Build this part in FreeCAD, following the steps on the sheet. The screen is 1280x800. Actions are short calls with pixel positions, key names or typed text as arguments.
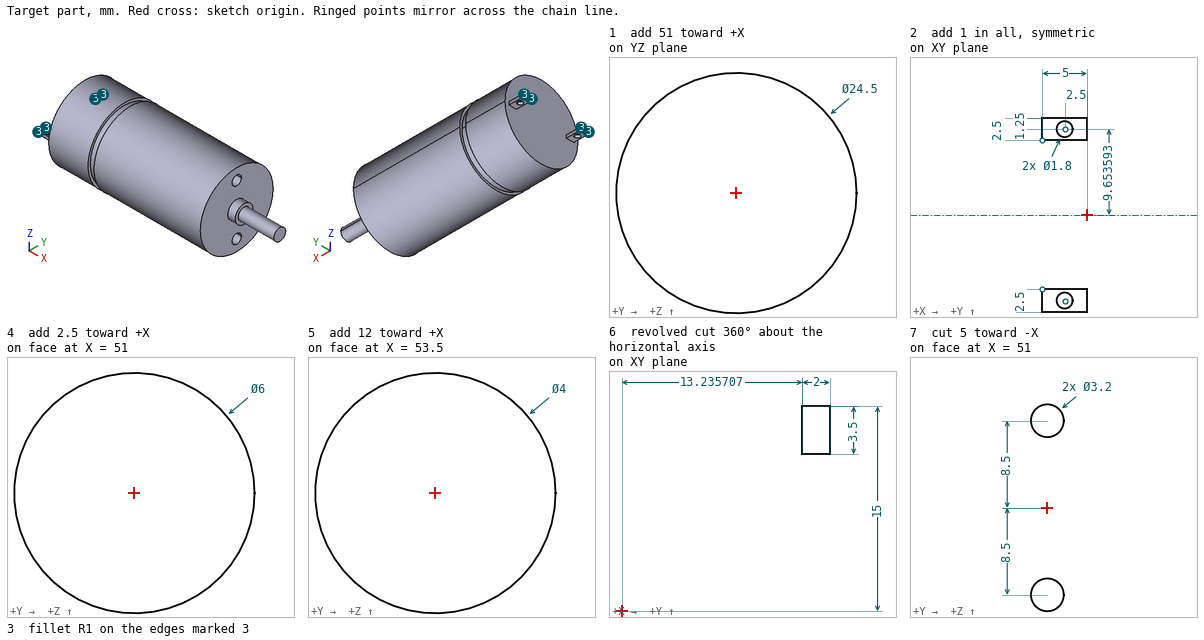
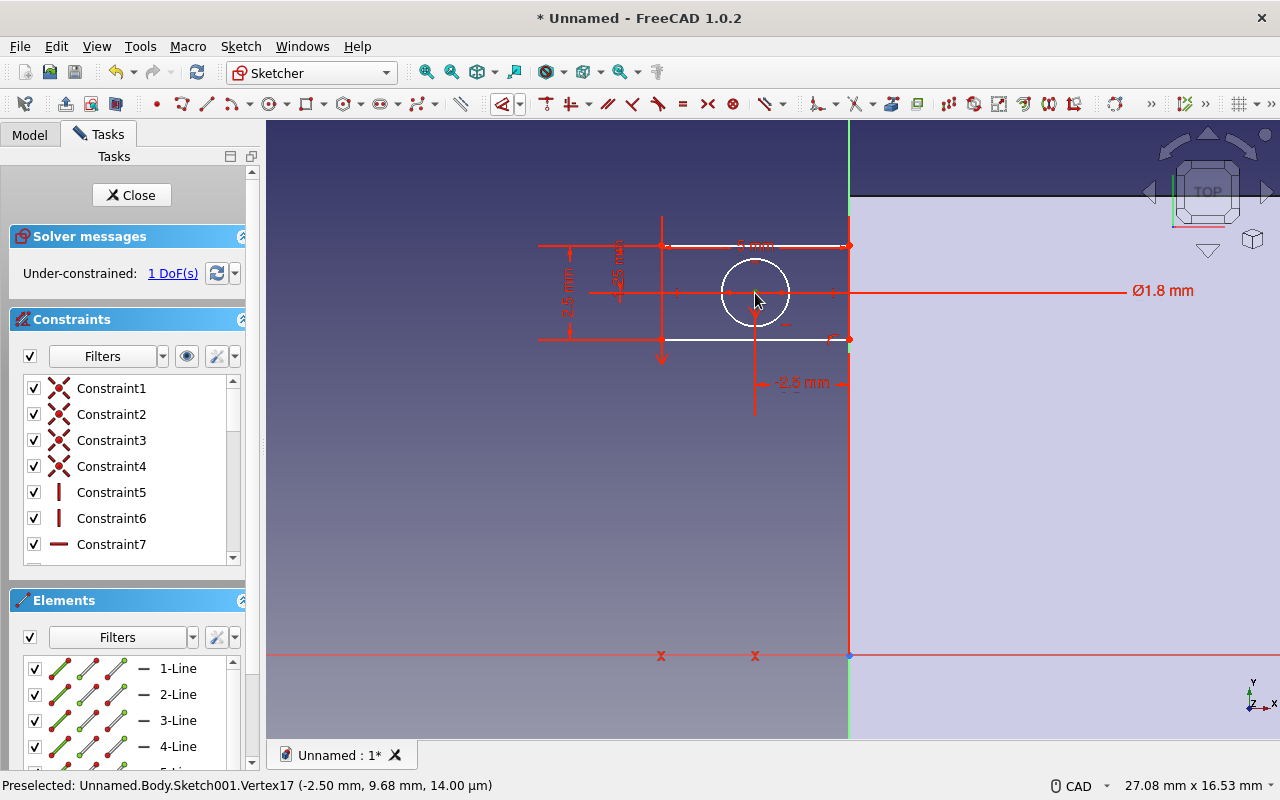
click(520, 104)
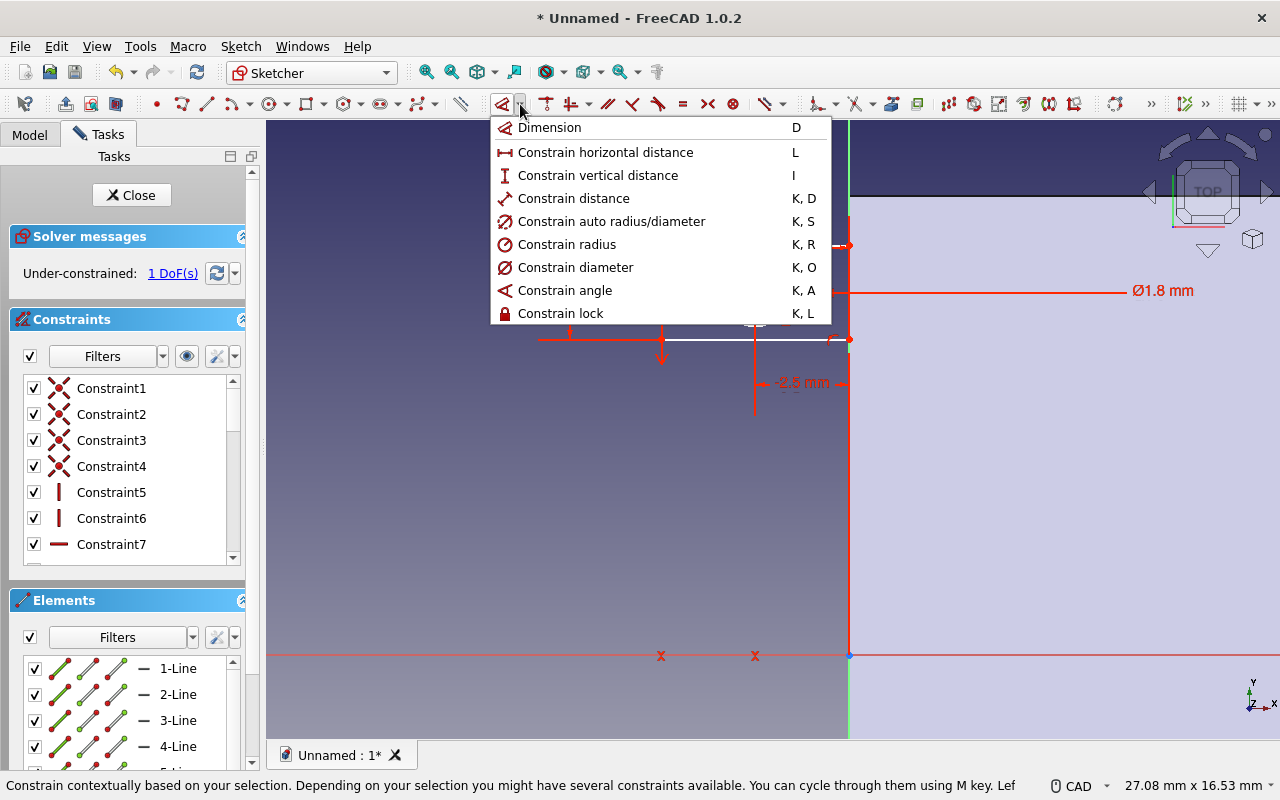
click(661, 176)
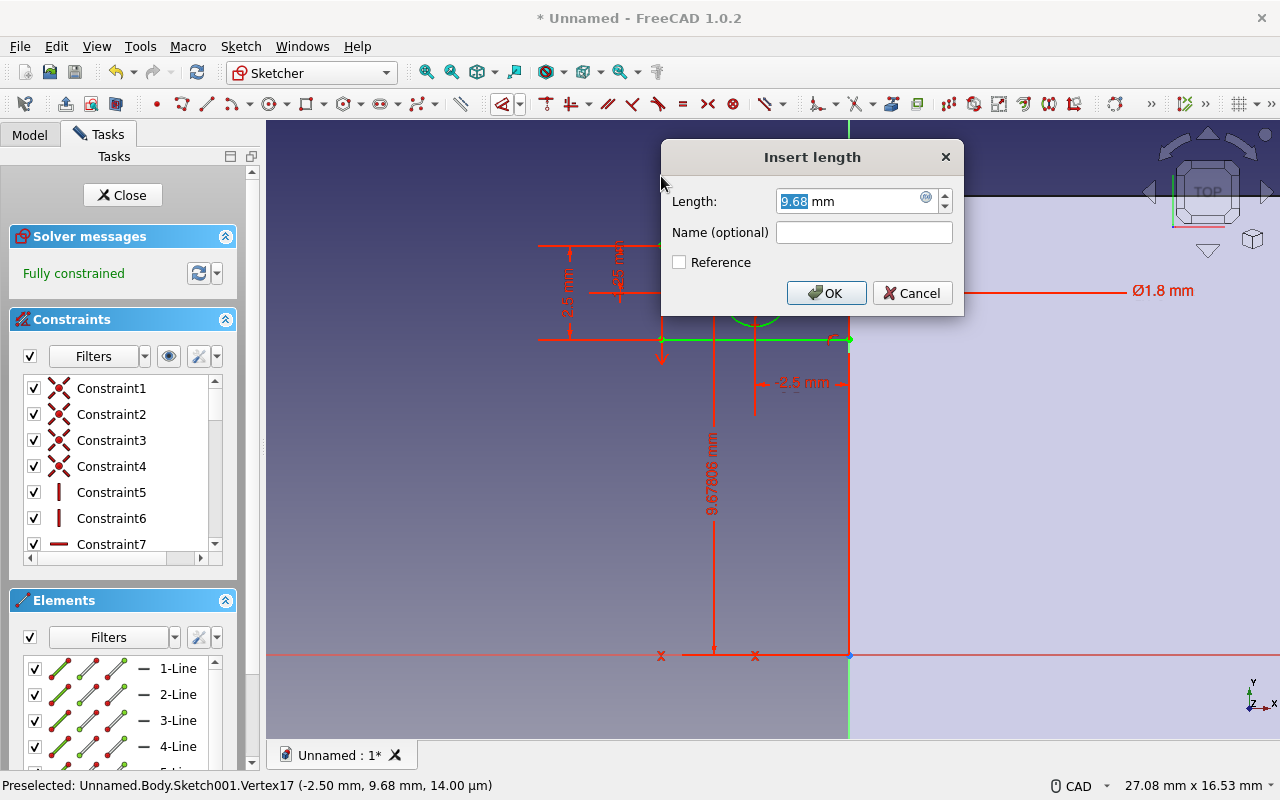
text(9.653593)
key(Return)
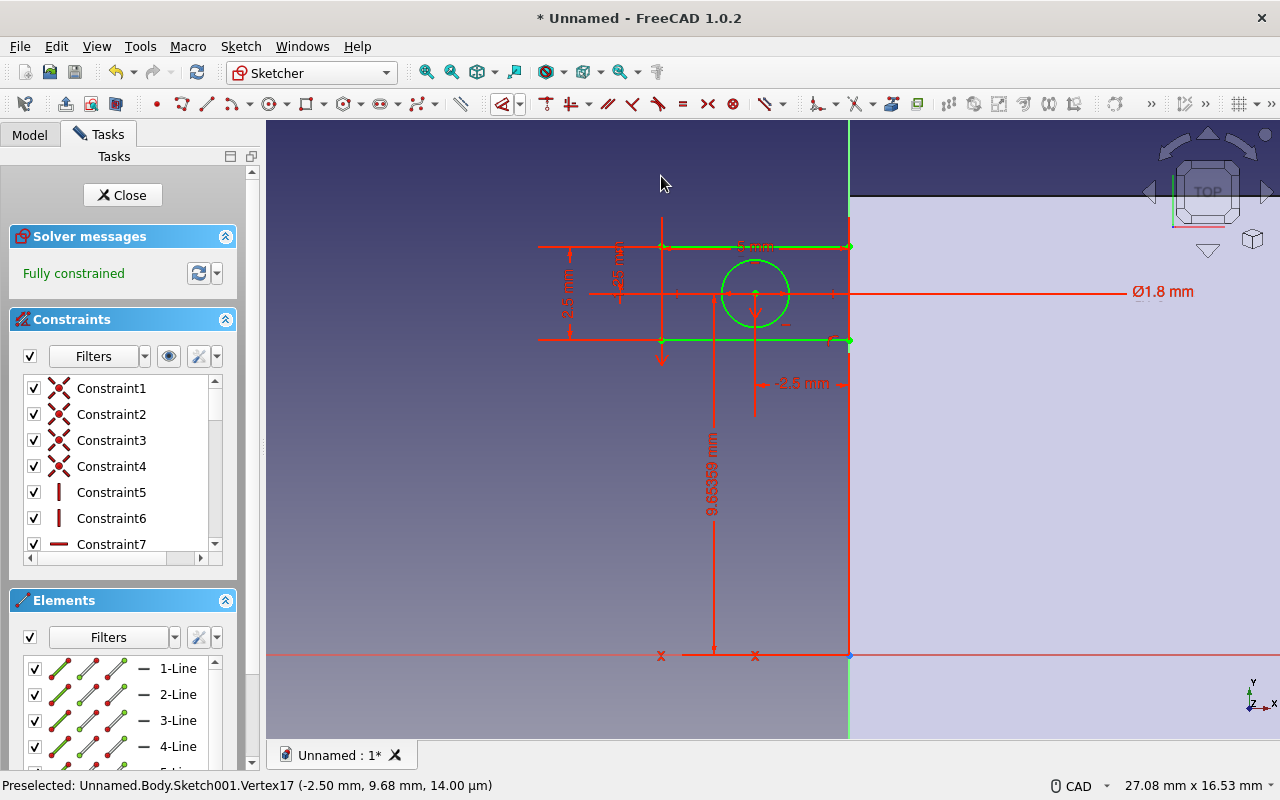
click(123, 195)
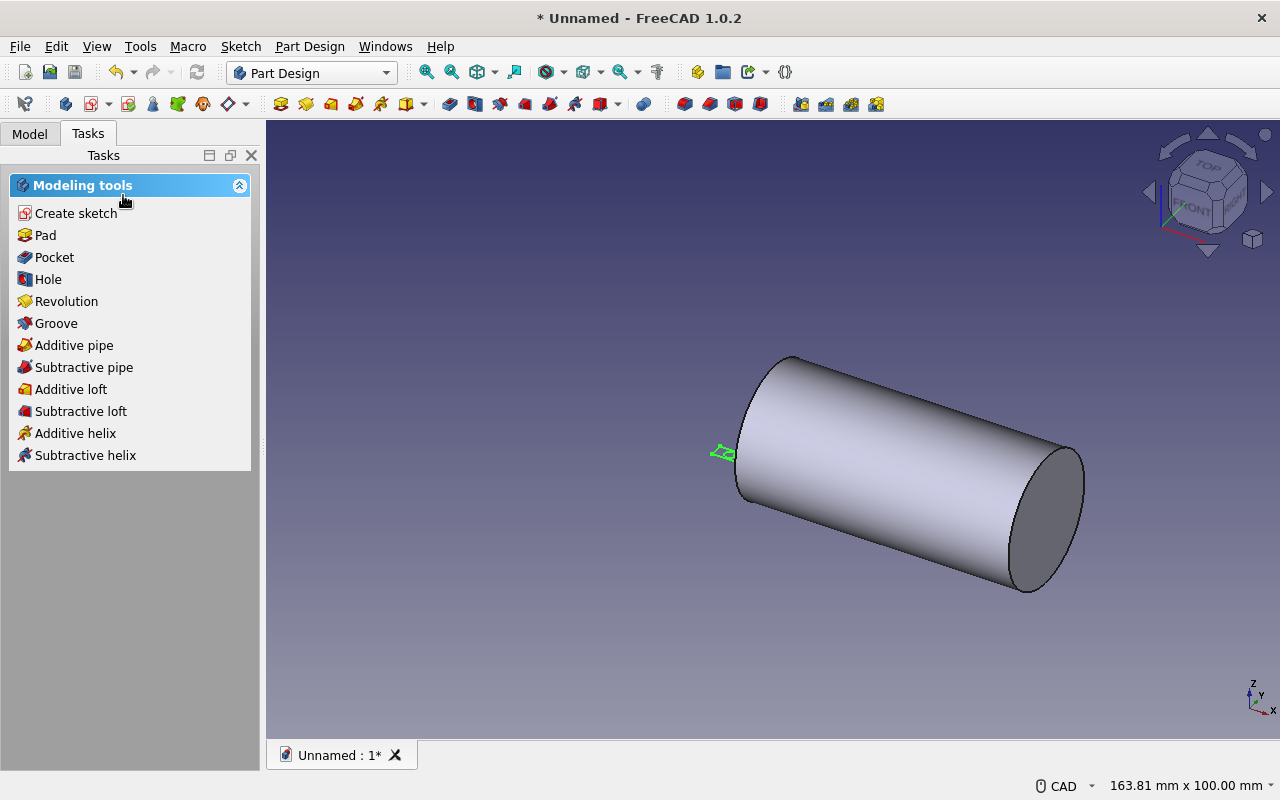
click(281, 104)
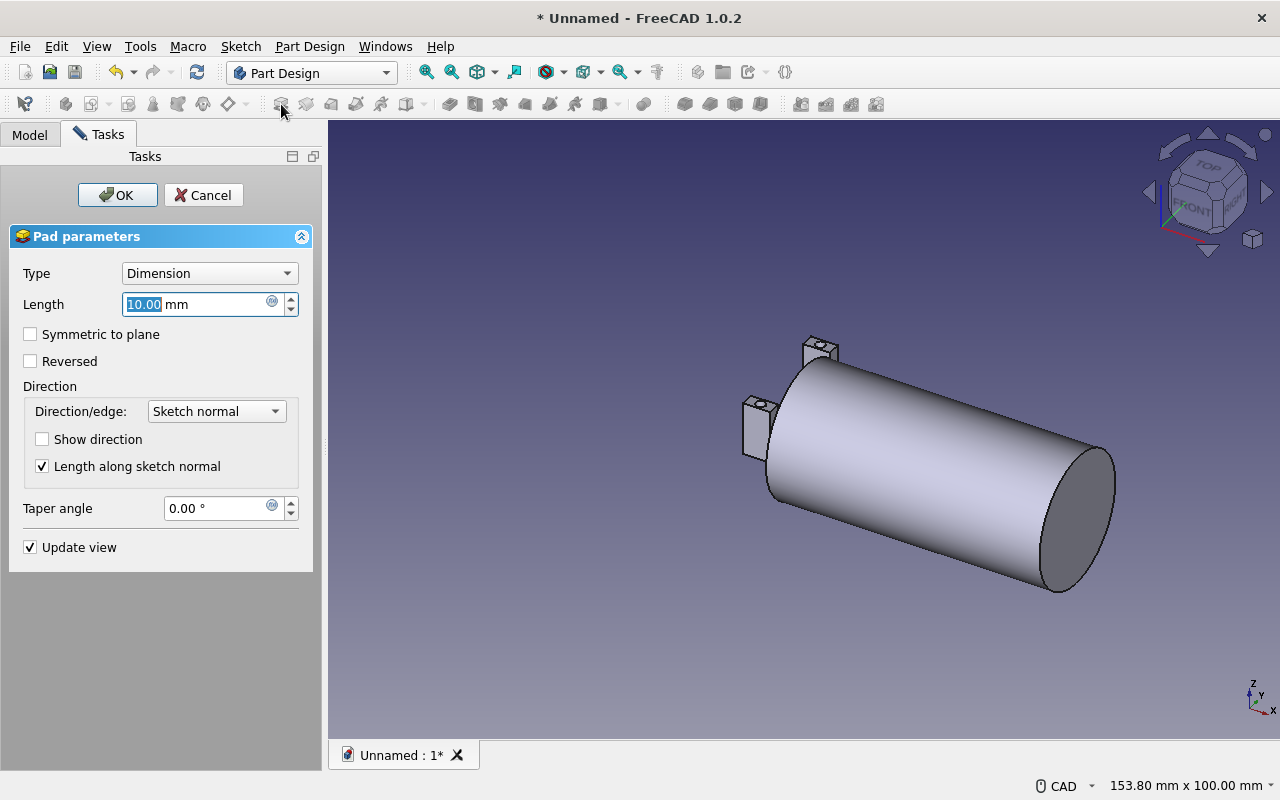
text(1)
key(Tab)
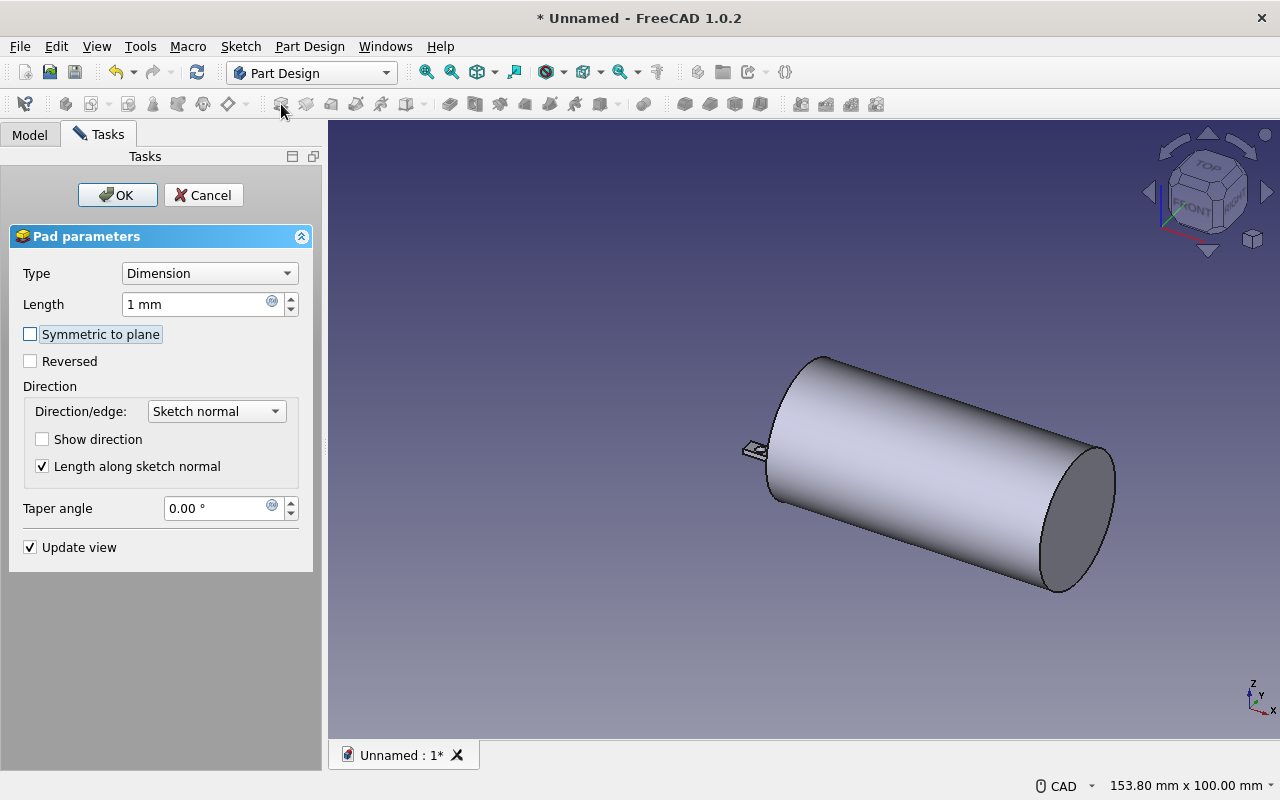
click(31, 334)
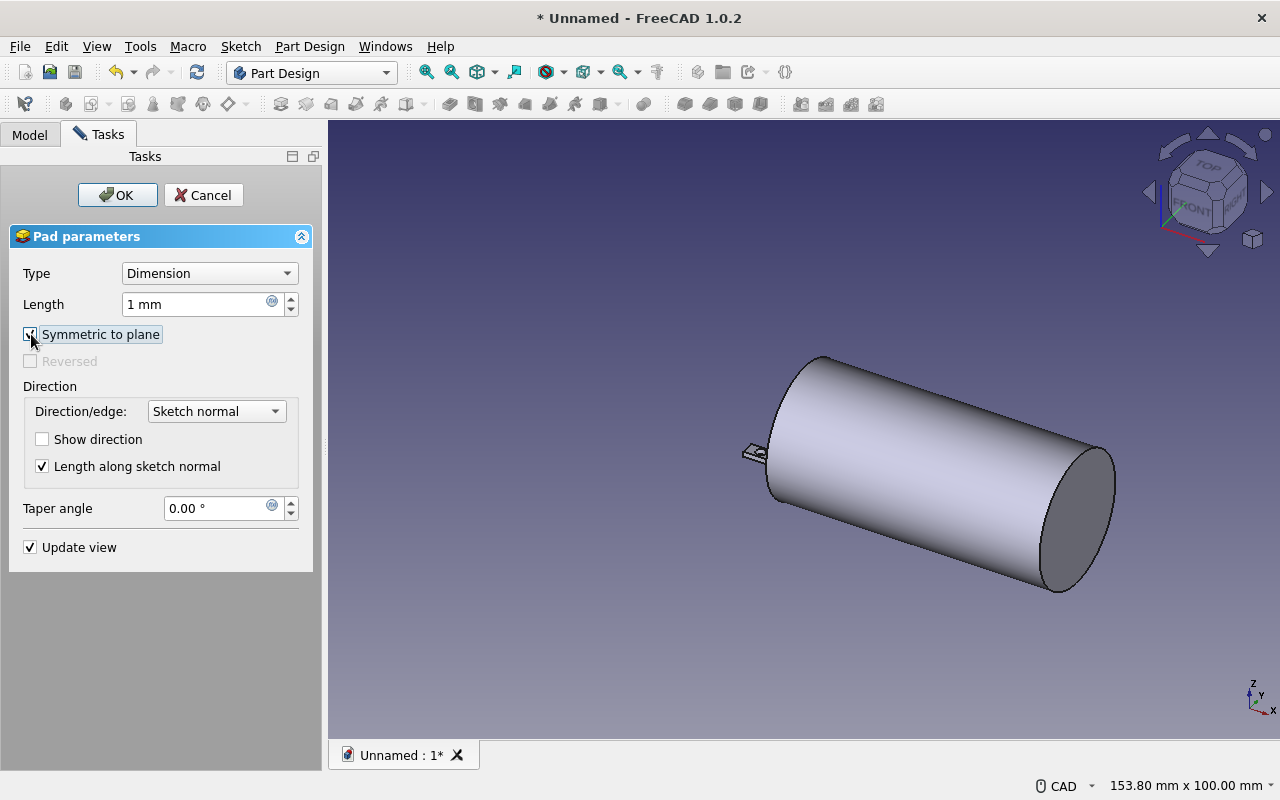
click(118, 195)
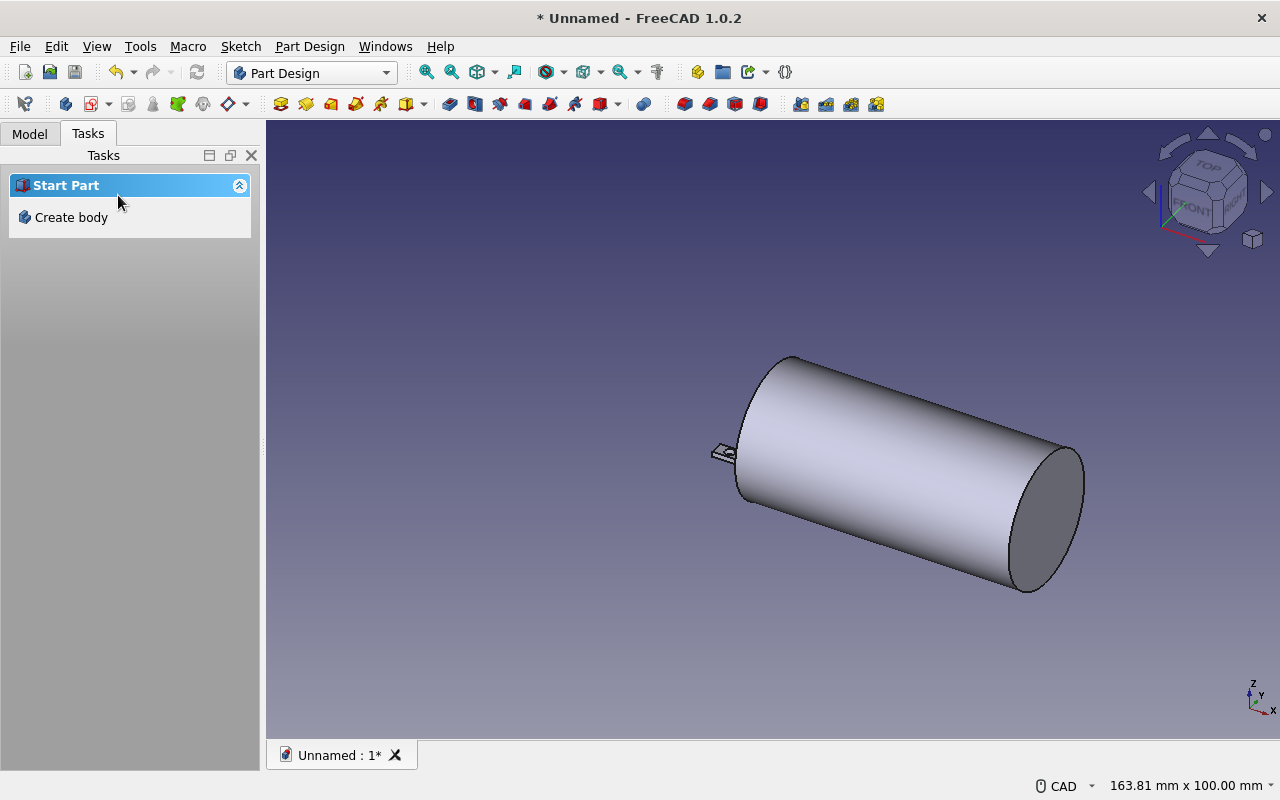
scroll(772, 394, up, 10)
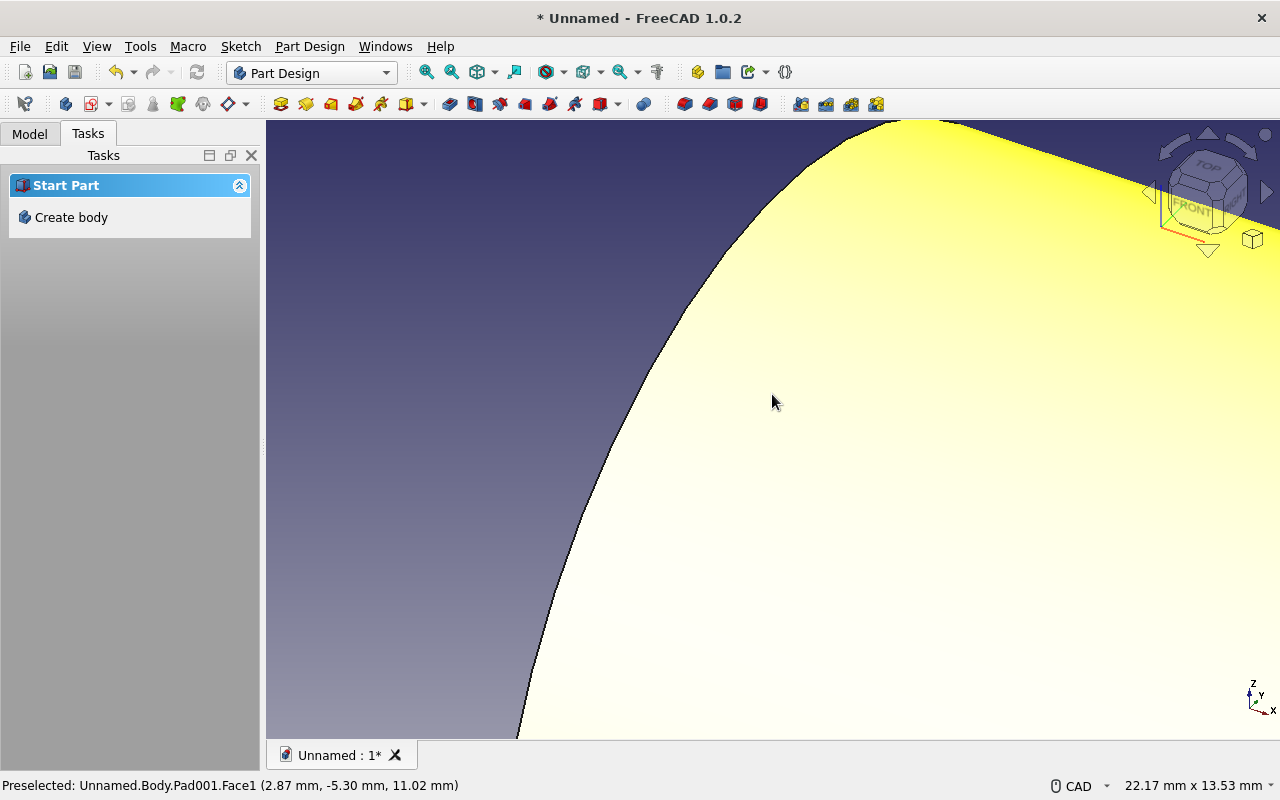
click(427, 72)